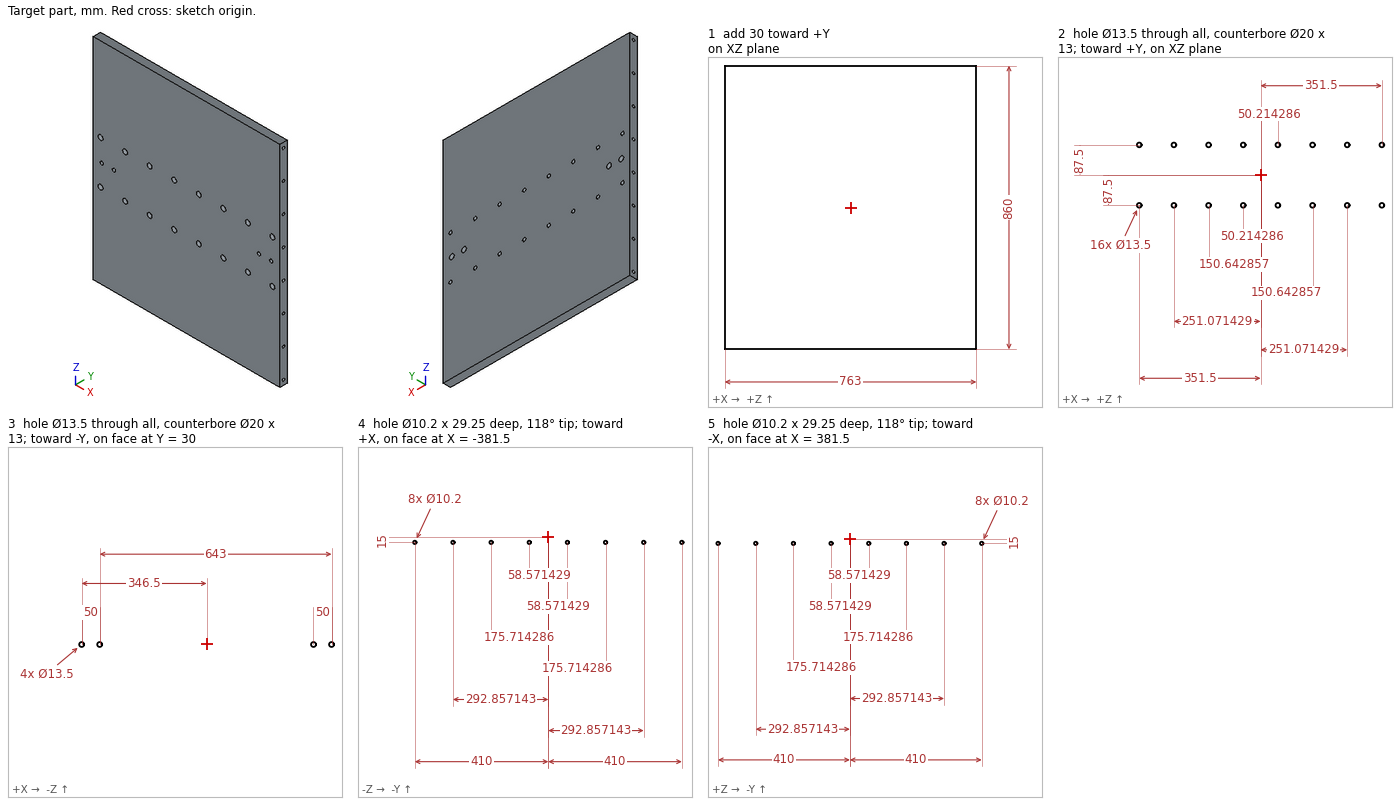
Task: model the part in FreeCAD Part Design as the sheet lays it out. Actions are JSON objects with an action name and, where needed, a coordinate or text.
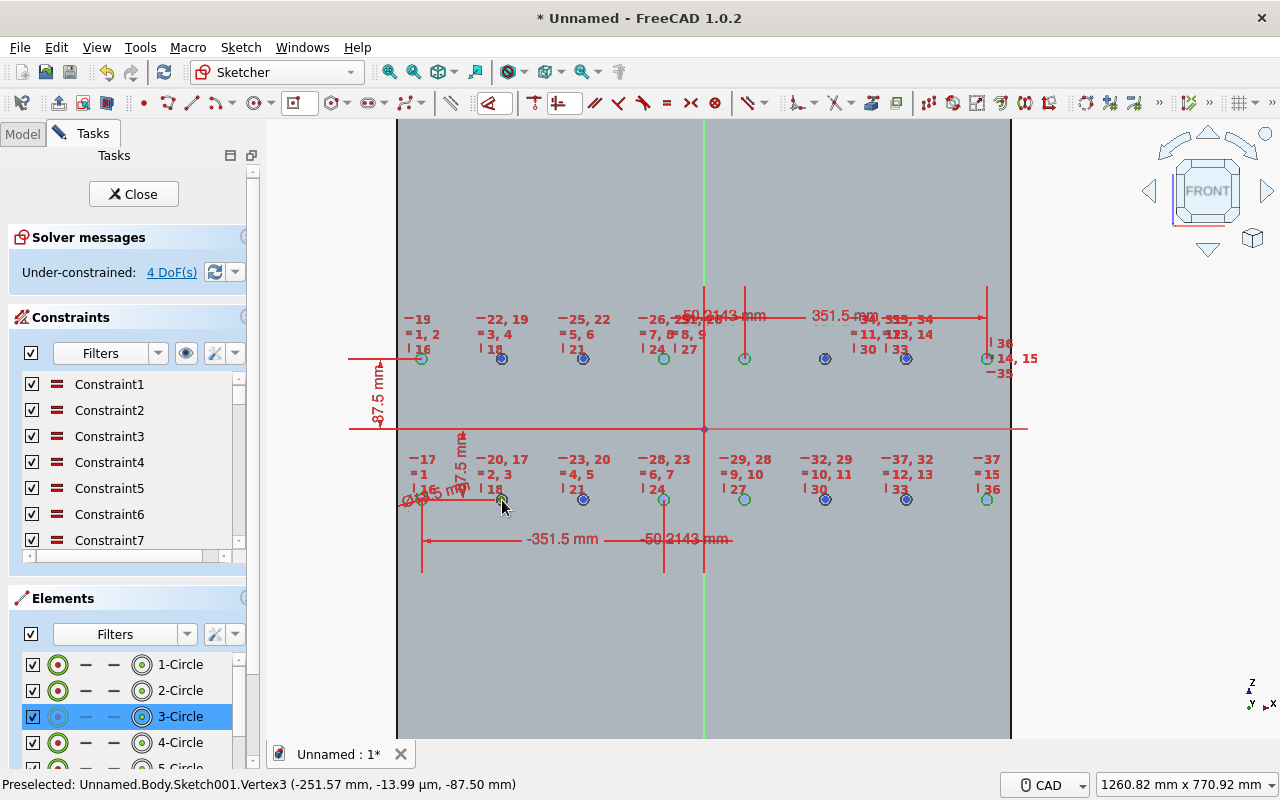
{"action": "left_click", "coordinate": [506, 104]}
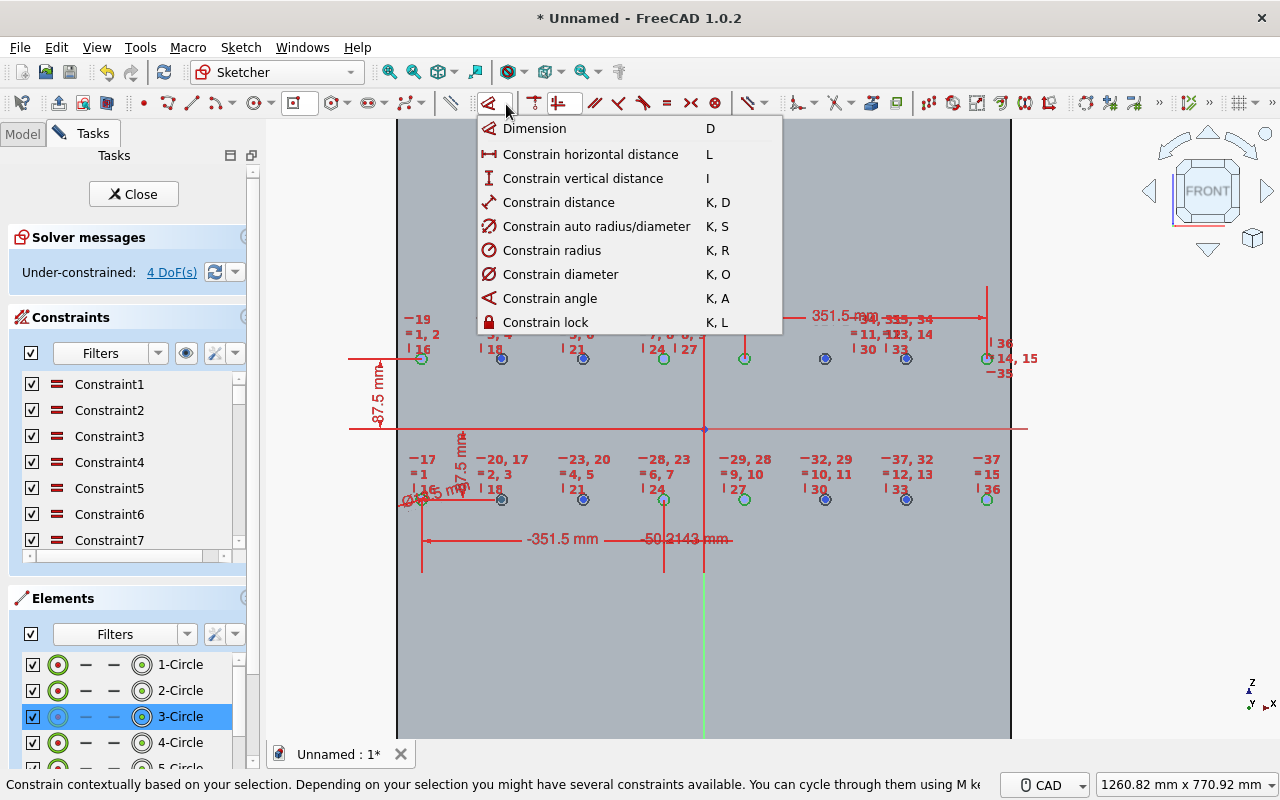
{"action": "left_click", "coordinate": [630, 154]}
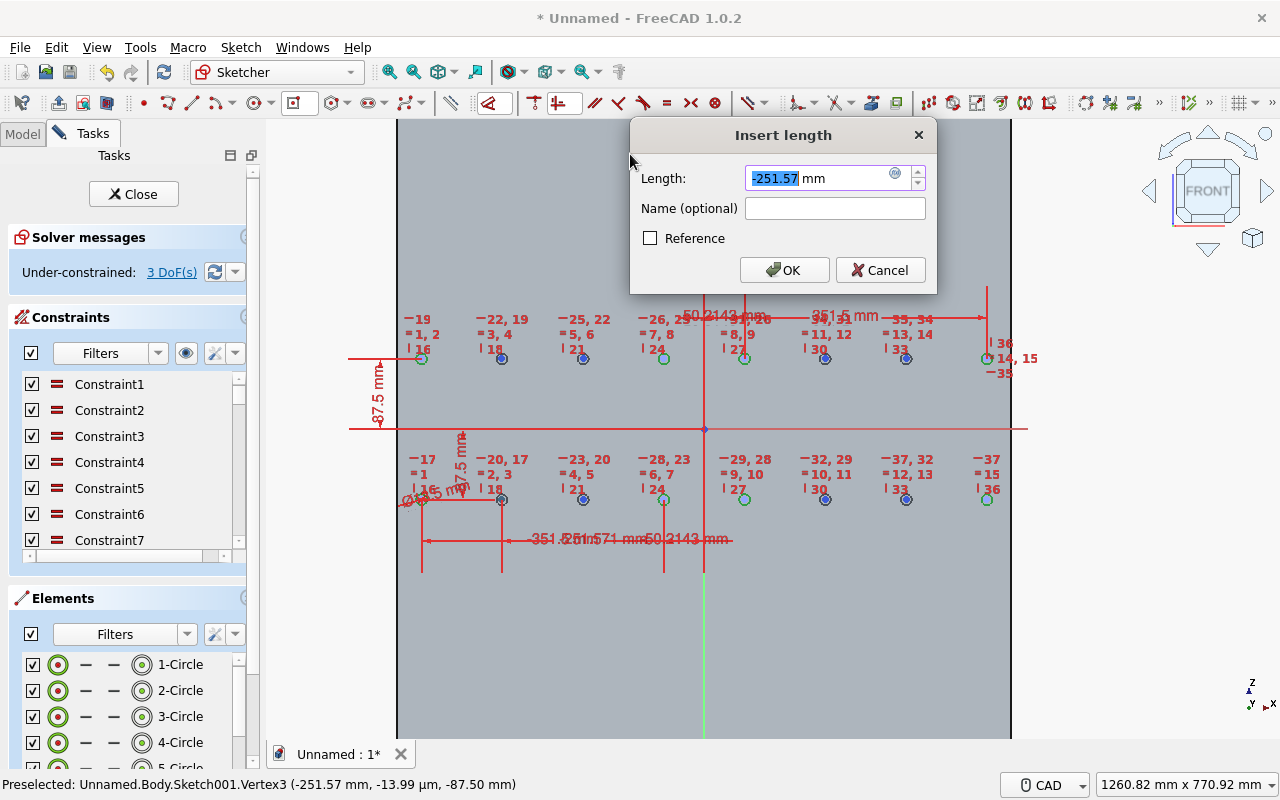
{"action": "type", "text": "-251.071429"}
{"action": "key", "text": "Return"}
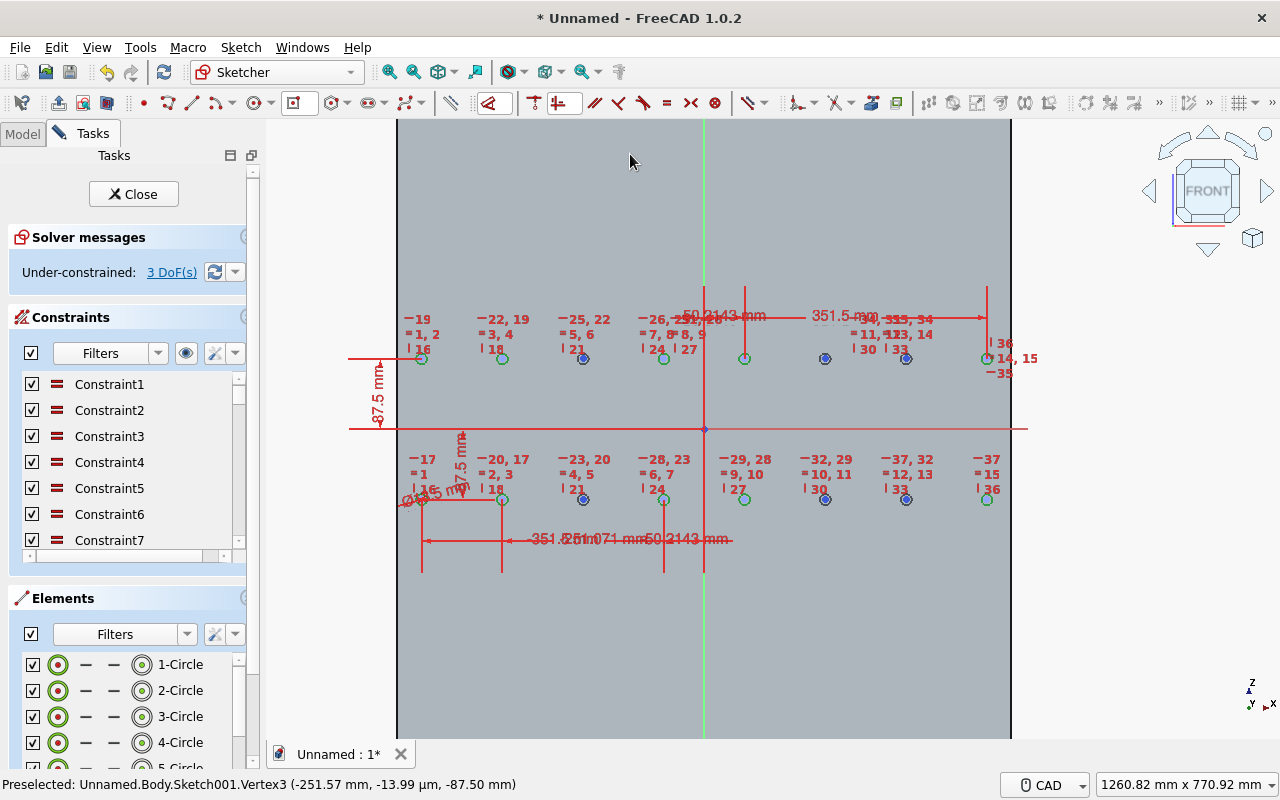
{"action": "left_click", "coordinate": [583, 500]}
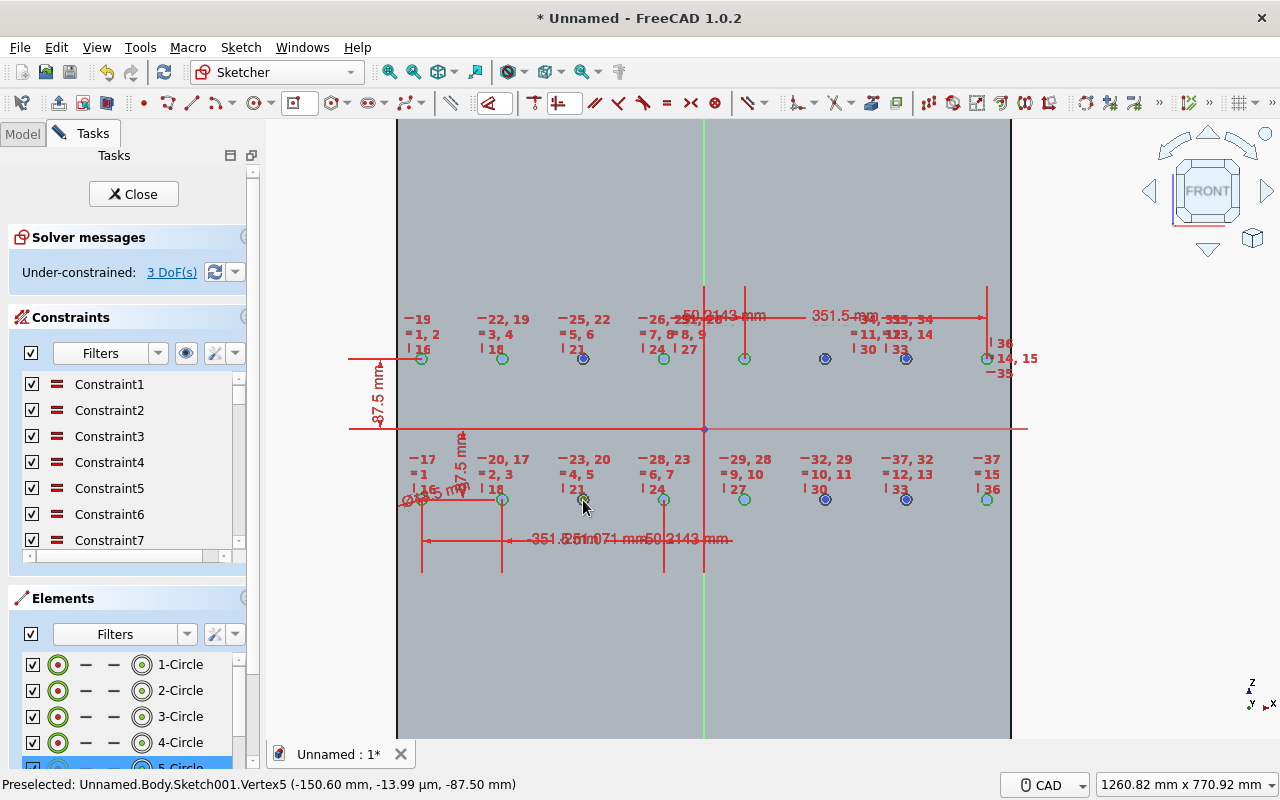
{"action": "left_click", "coordinate": [506, 104]}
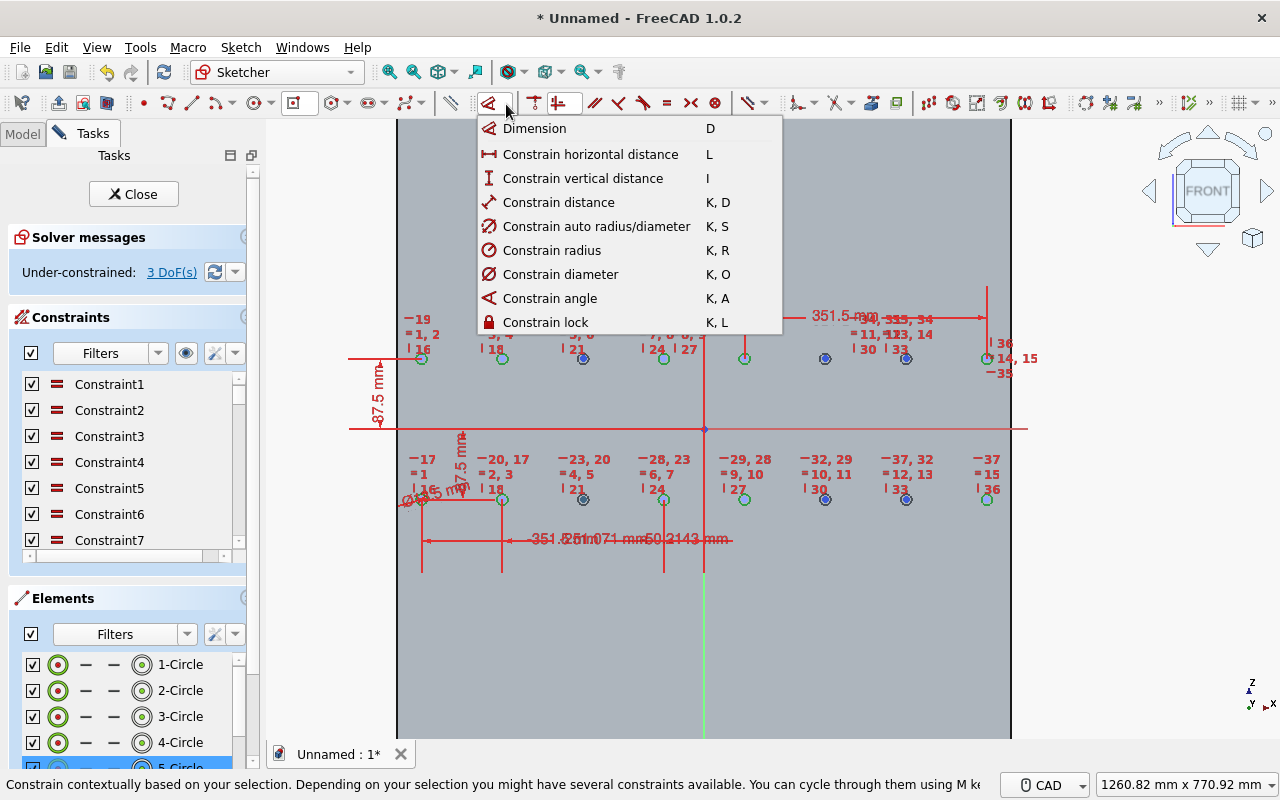
{"action": "left_click", "coordinate": [630, 154]}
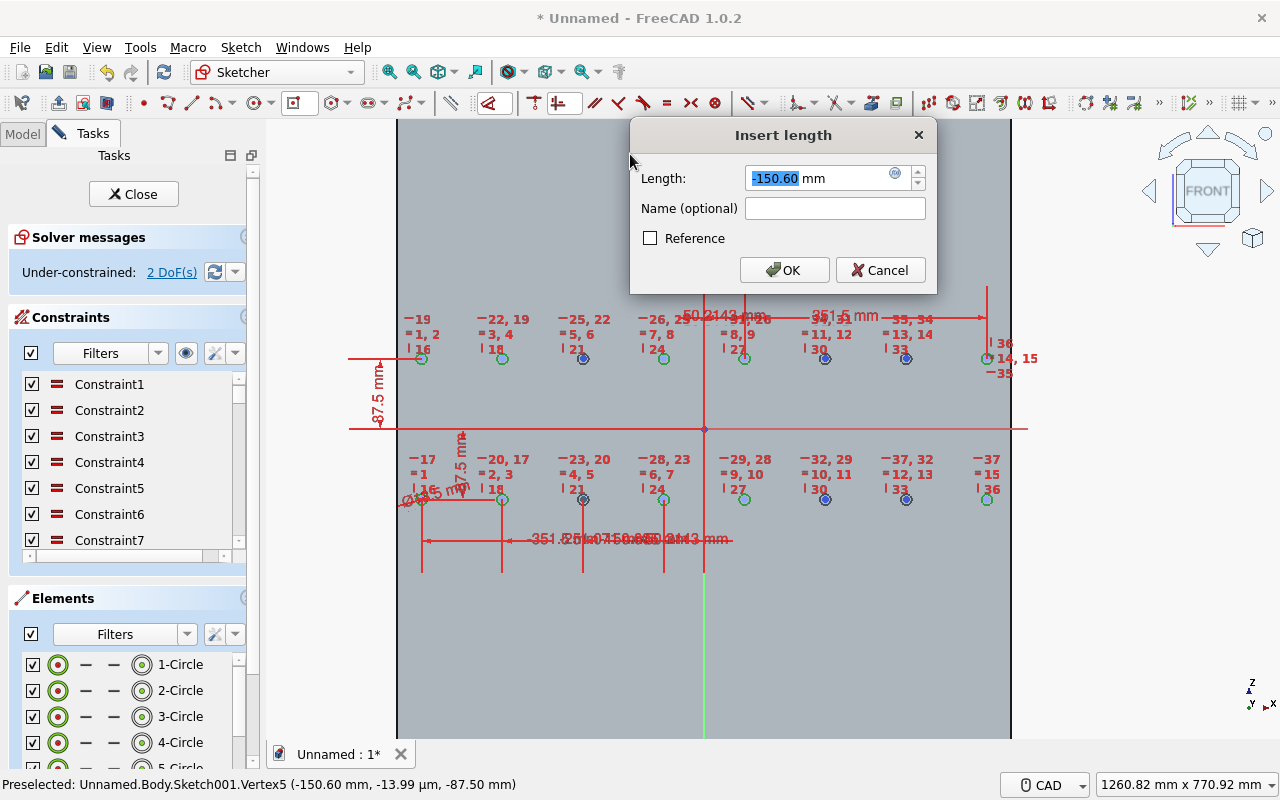
{"action": "type", "text": "-150.642857"}
{"action": "key", "text": "Return"}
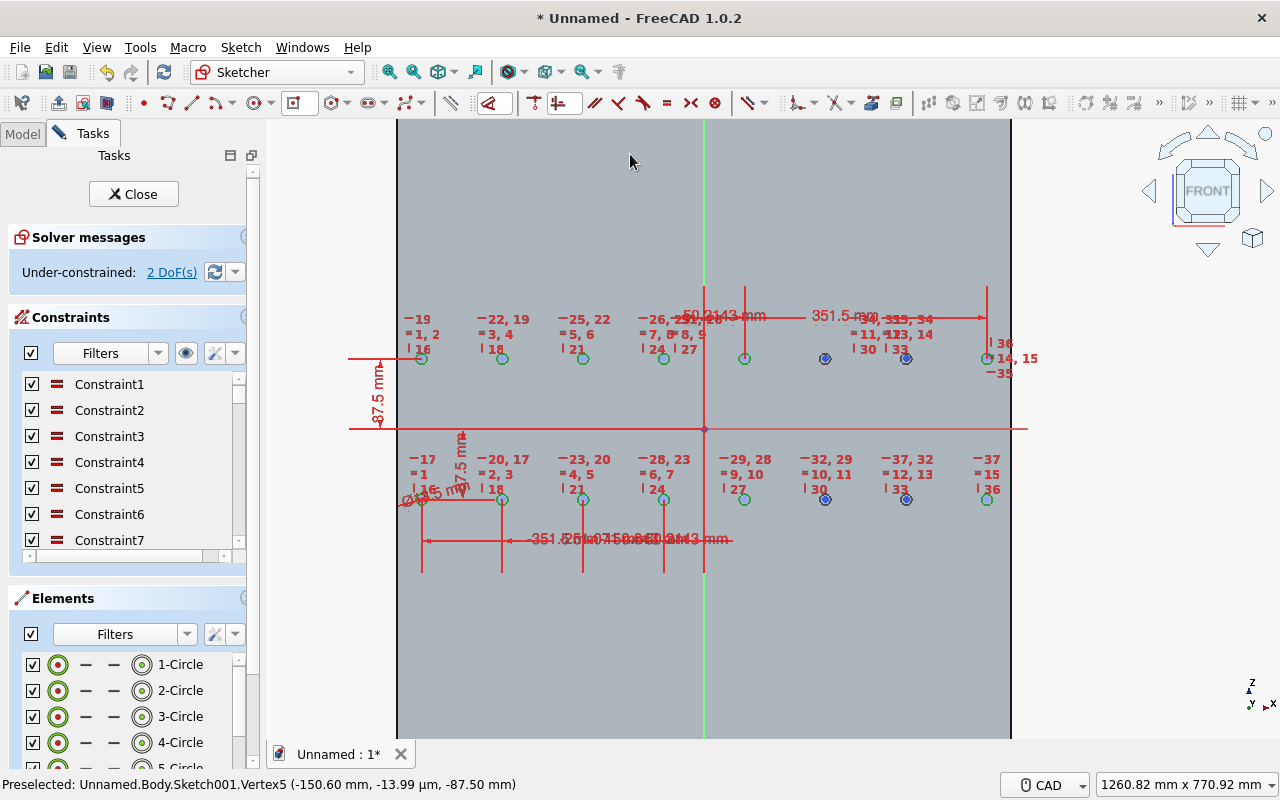
{"action": "left_click", "coordinate": [825, 500]}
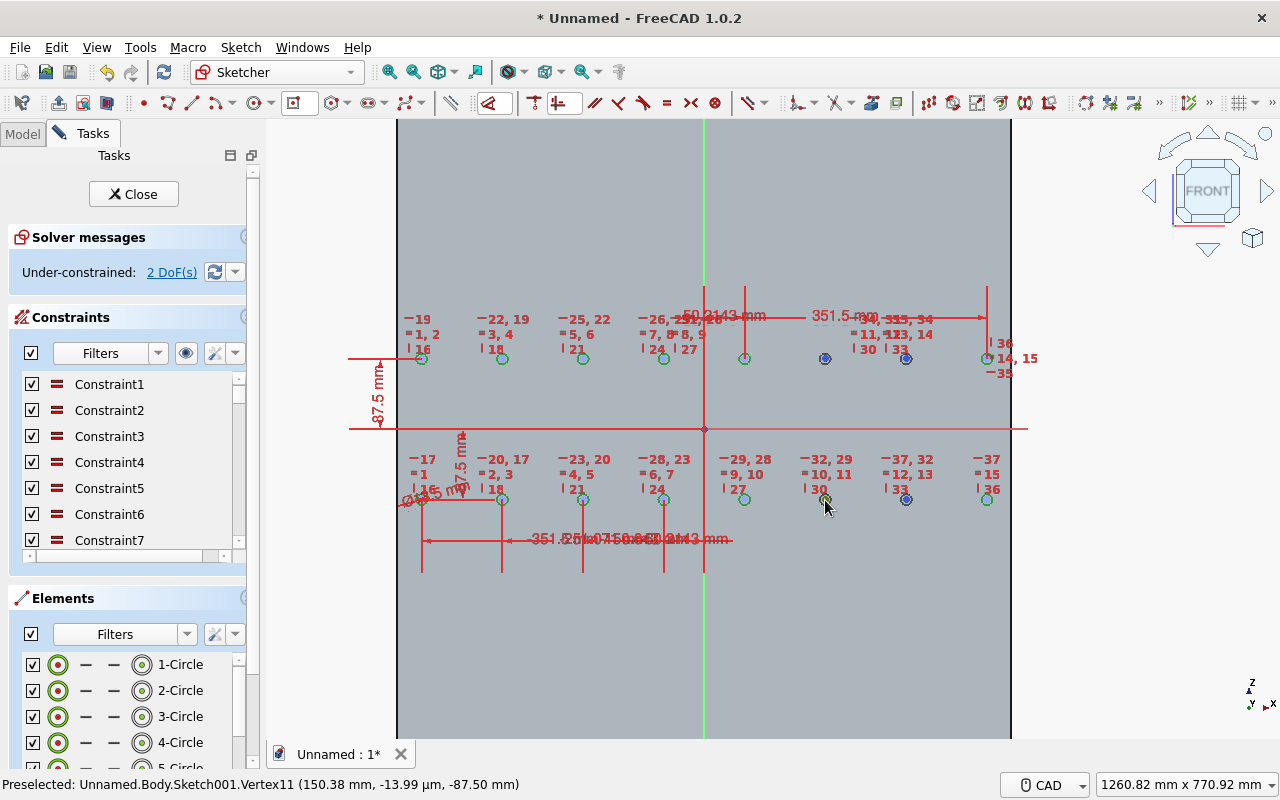
{"action": "key", "text": "l"}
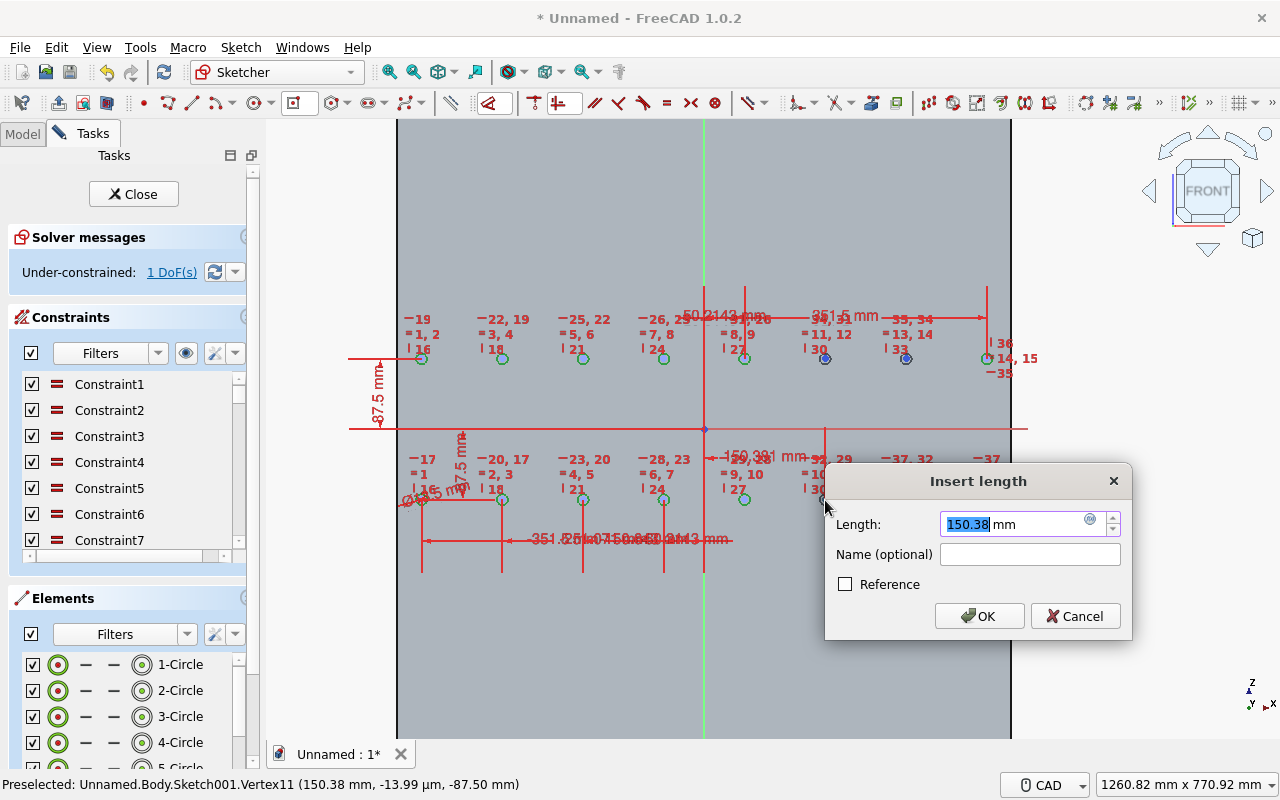
{"action": "type", "text": "150.642857"}
{"action": "key", "text": "Return"}